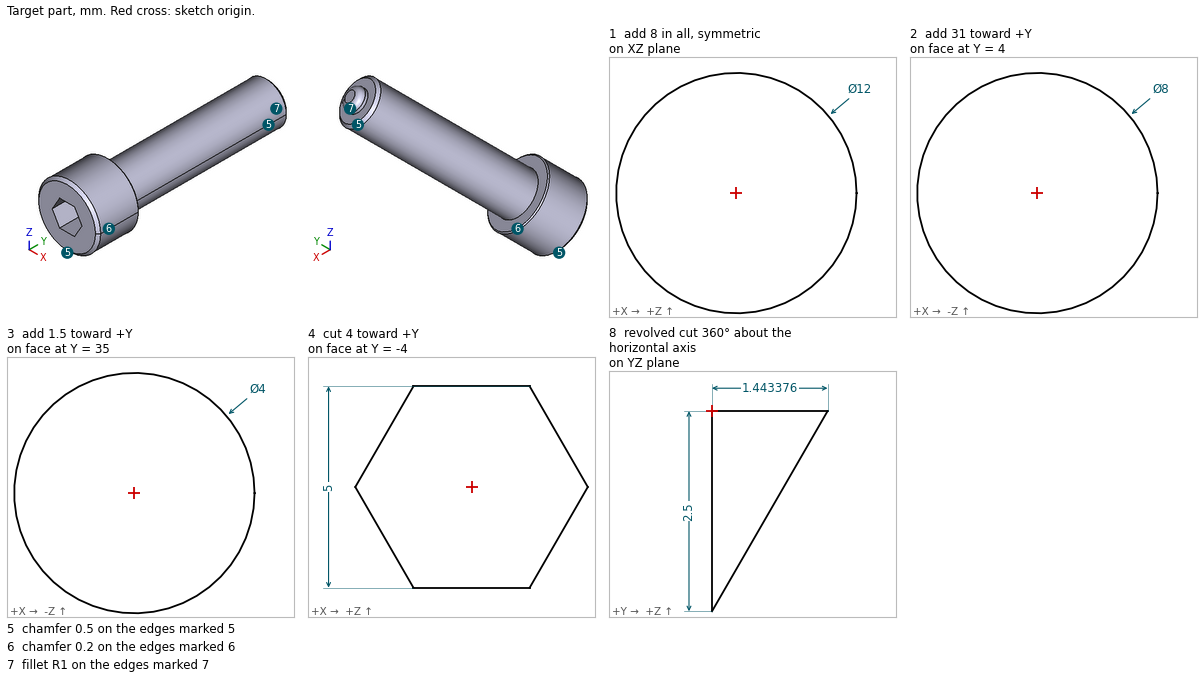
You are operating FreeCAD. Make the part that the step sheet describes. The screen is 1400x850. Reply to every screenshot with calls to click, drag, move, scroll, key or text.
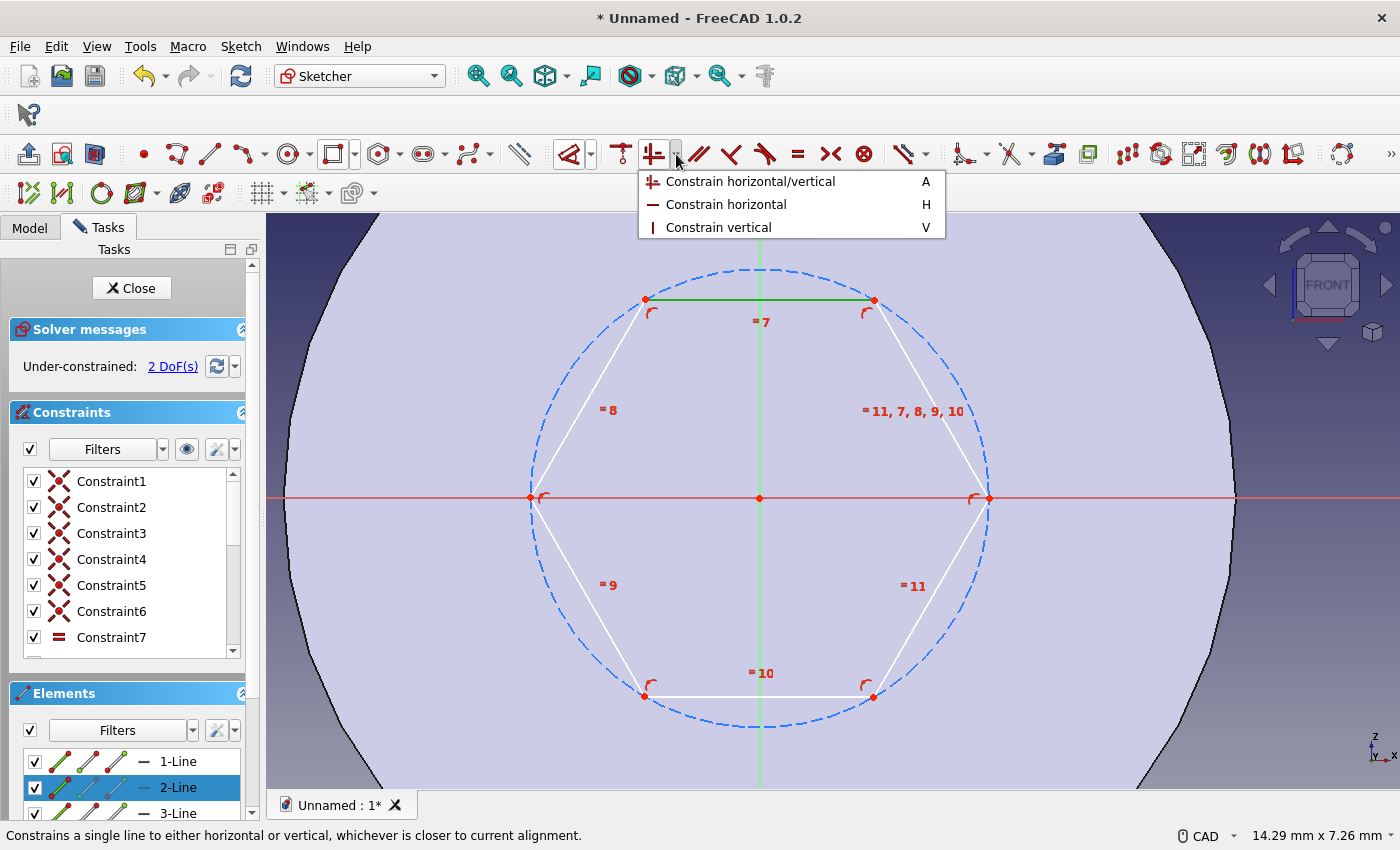
click(792, 204)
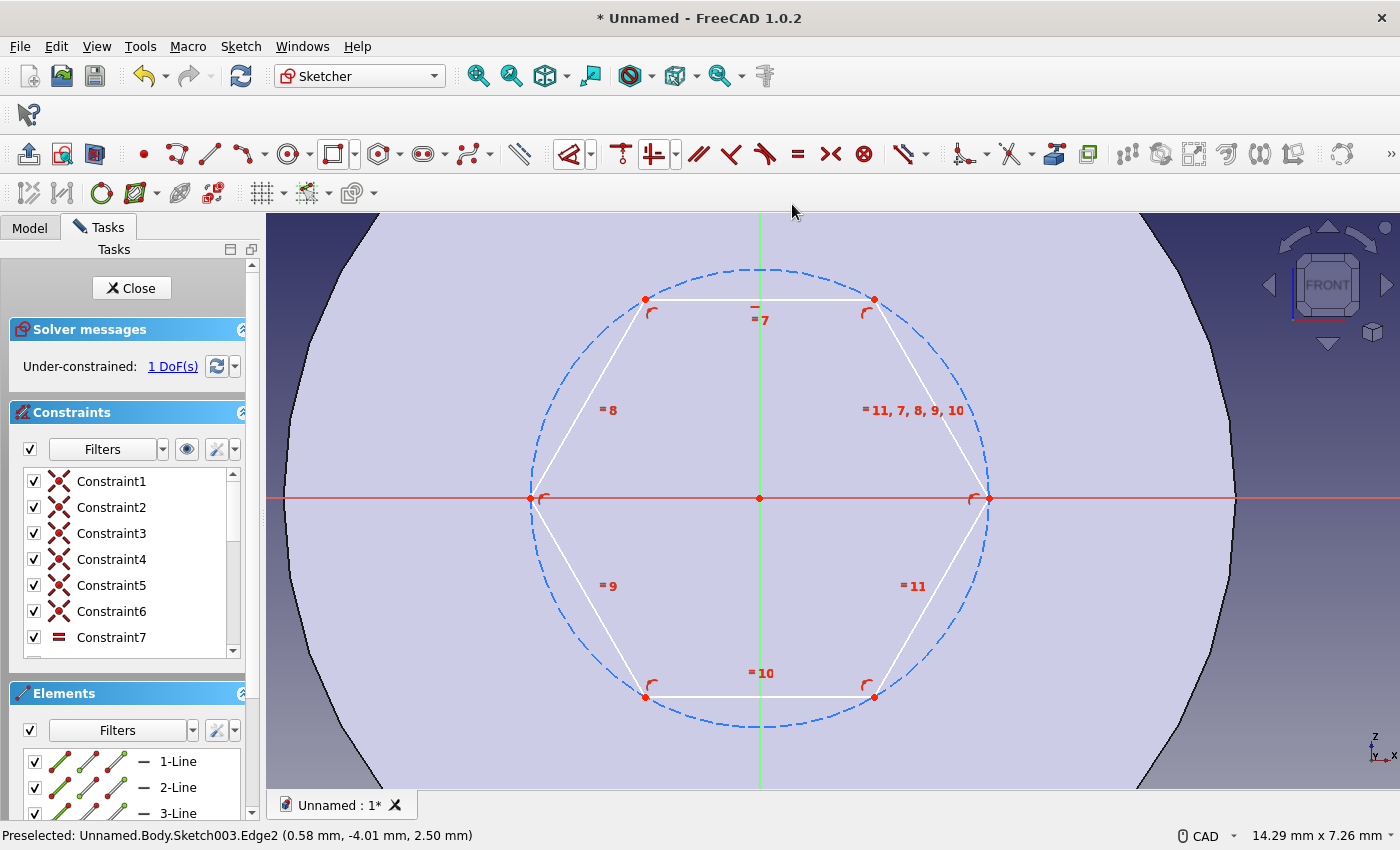
click(645, 697)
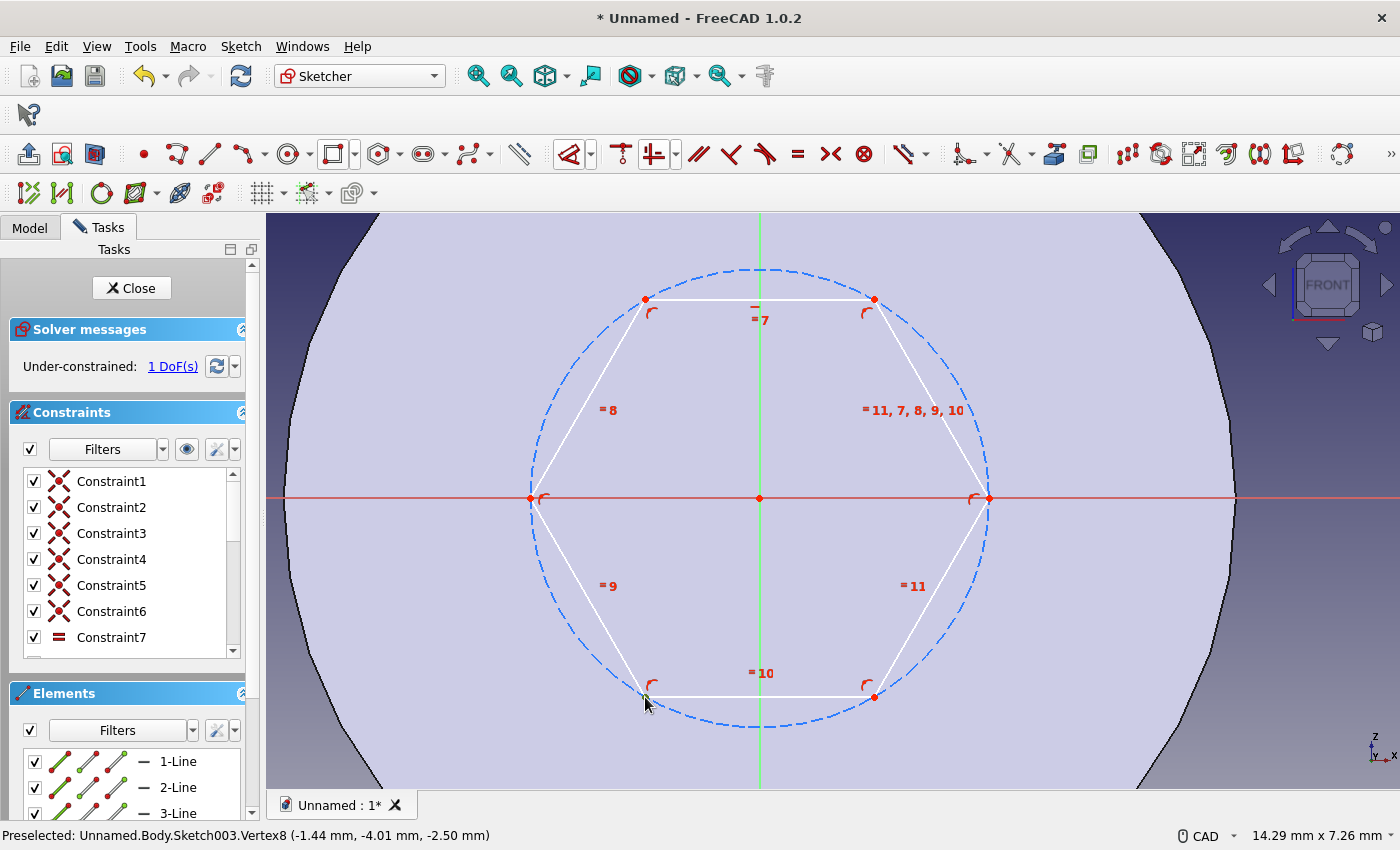
click(874, 300)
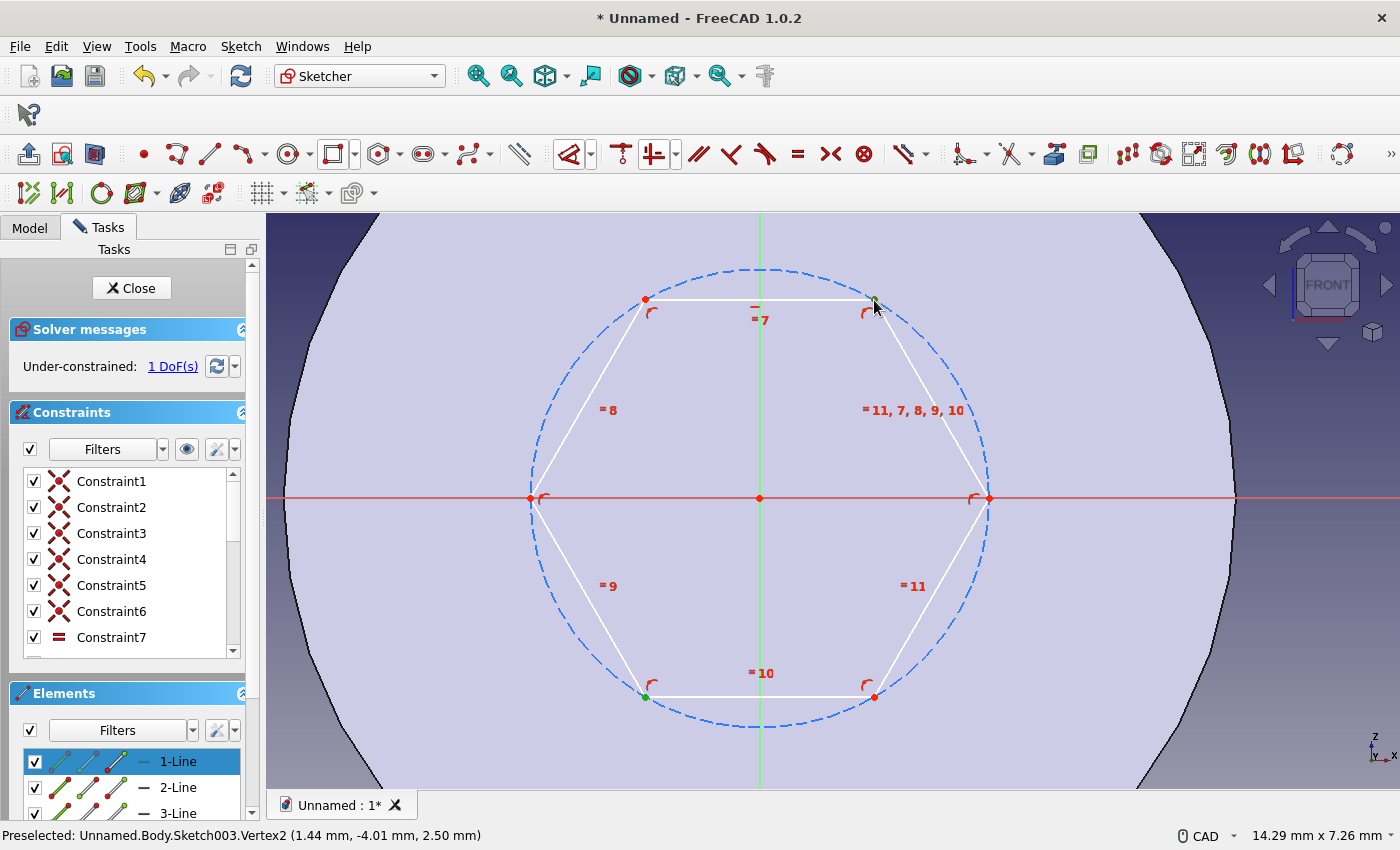
click(590, 154)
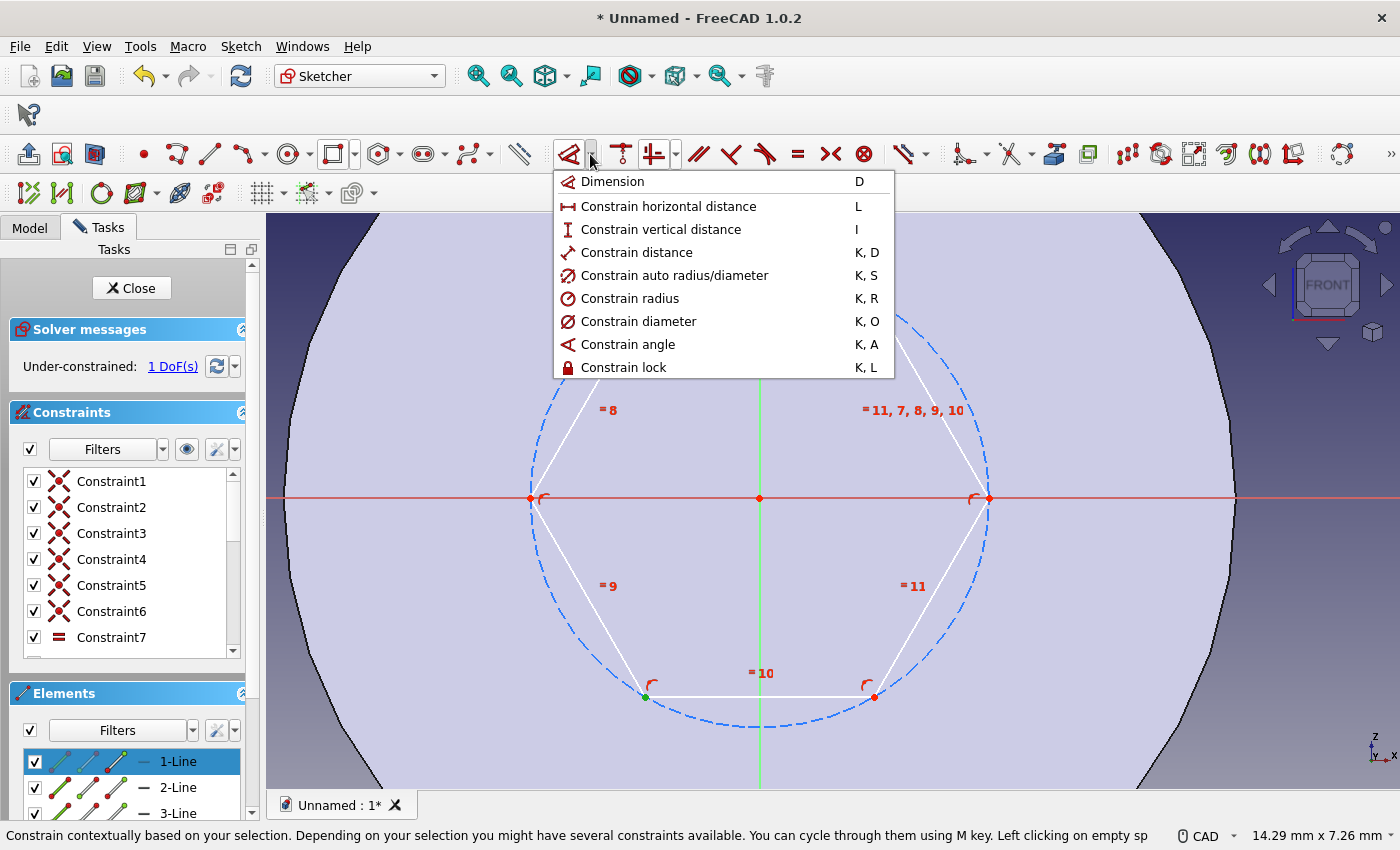
click(724, 230)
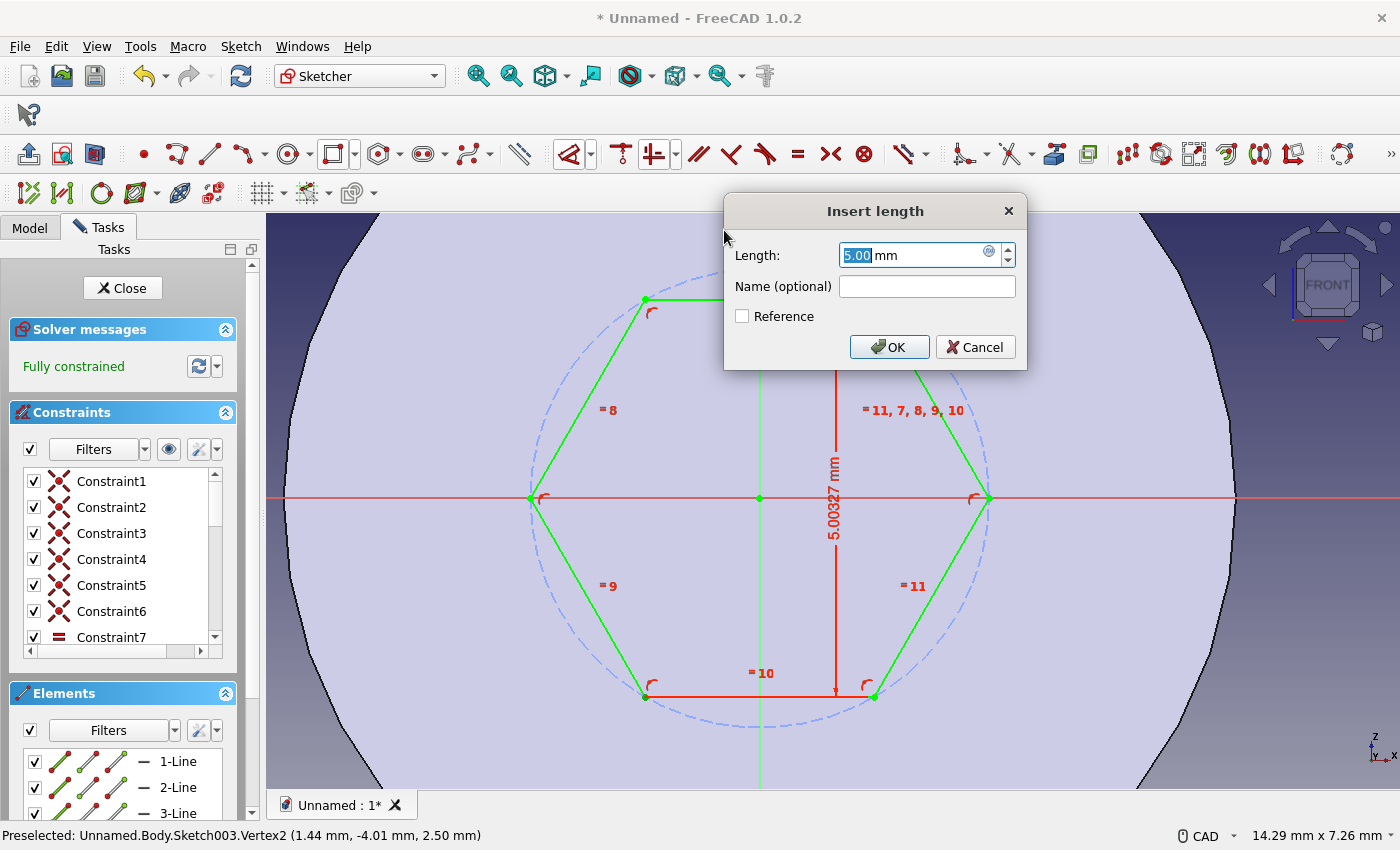
text(5)
key(Return)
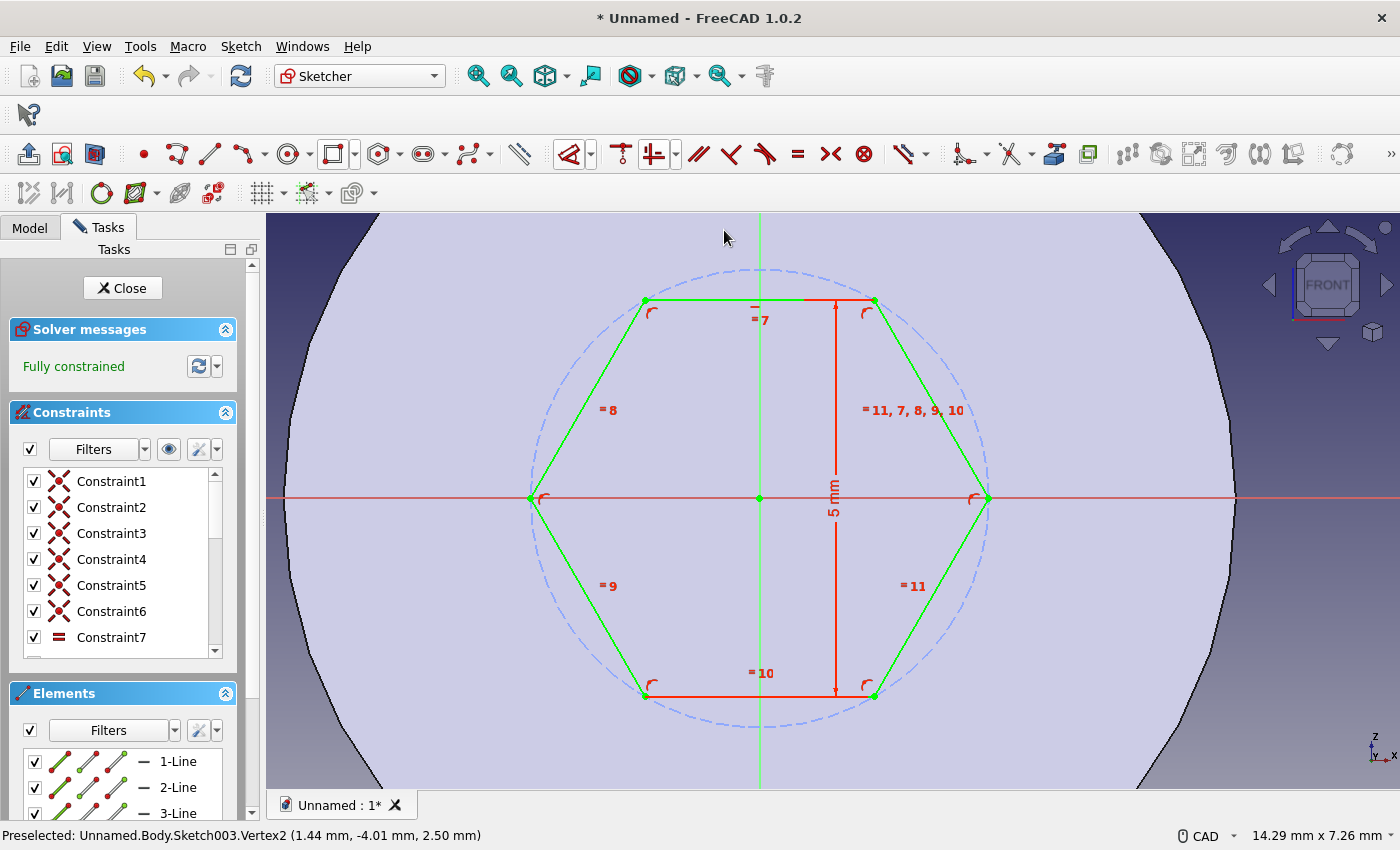
click(123, 288)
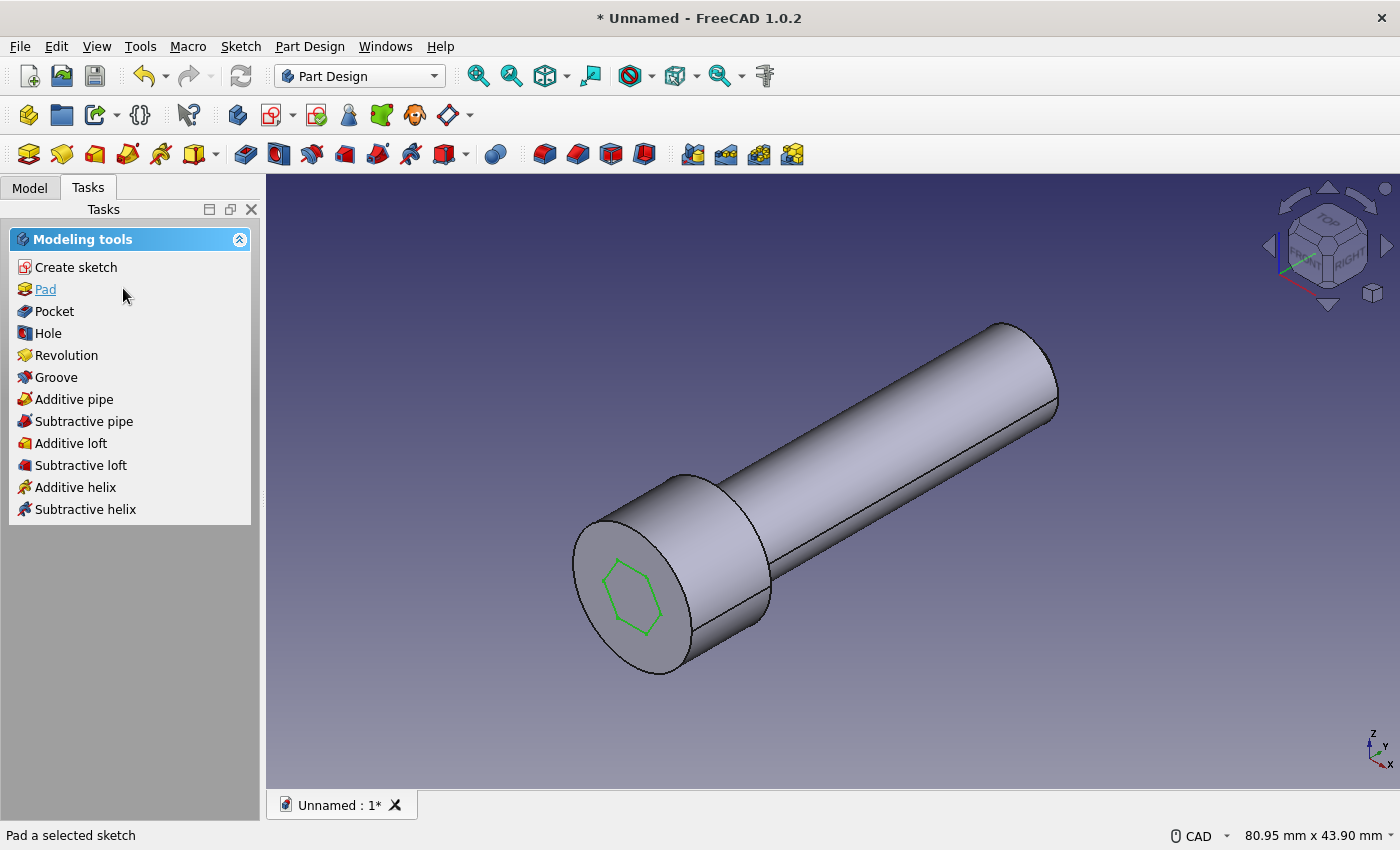
click(246, 154)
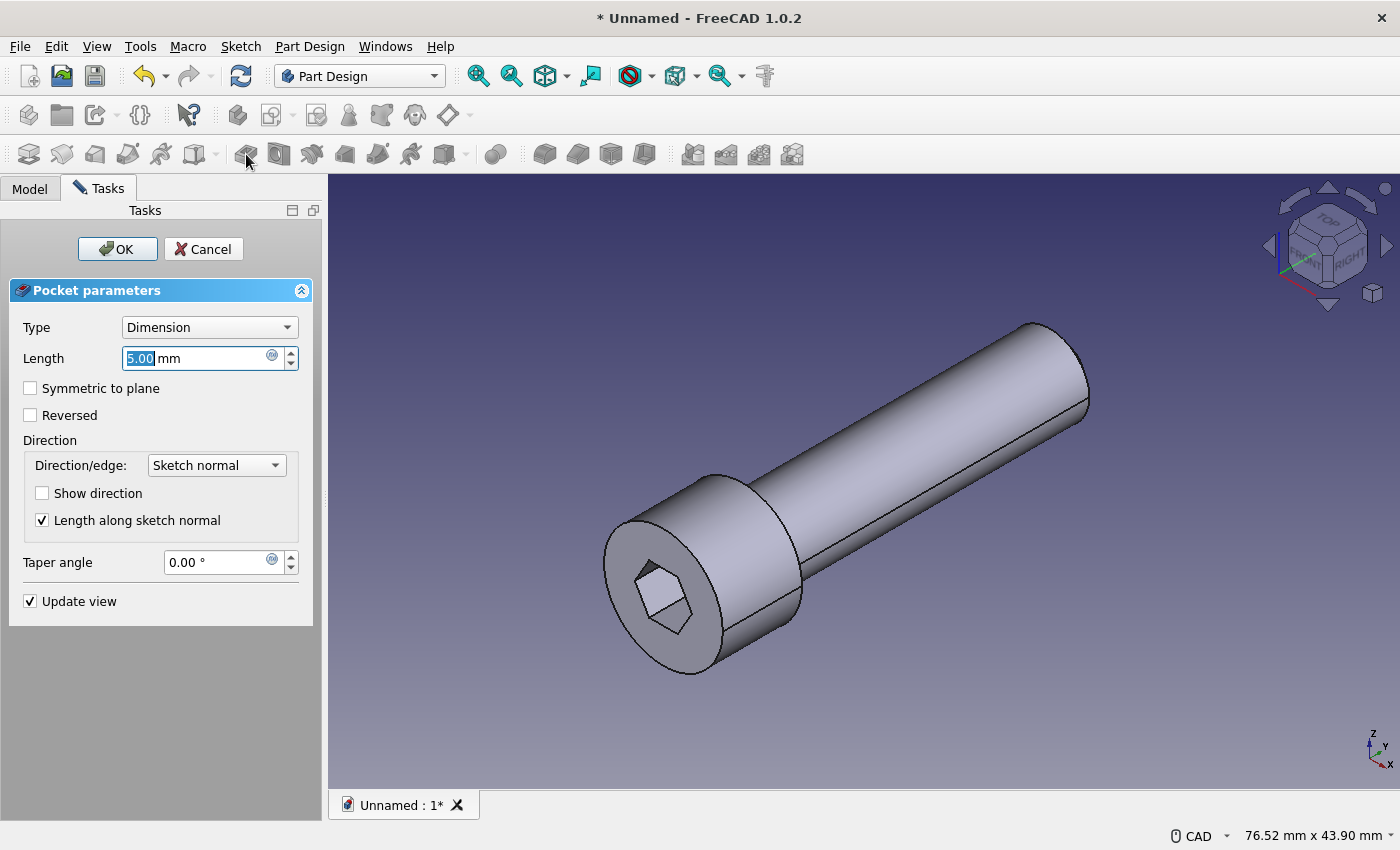
text(4)
key(Tab)